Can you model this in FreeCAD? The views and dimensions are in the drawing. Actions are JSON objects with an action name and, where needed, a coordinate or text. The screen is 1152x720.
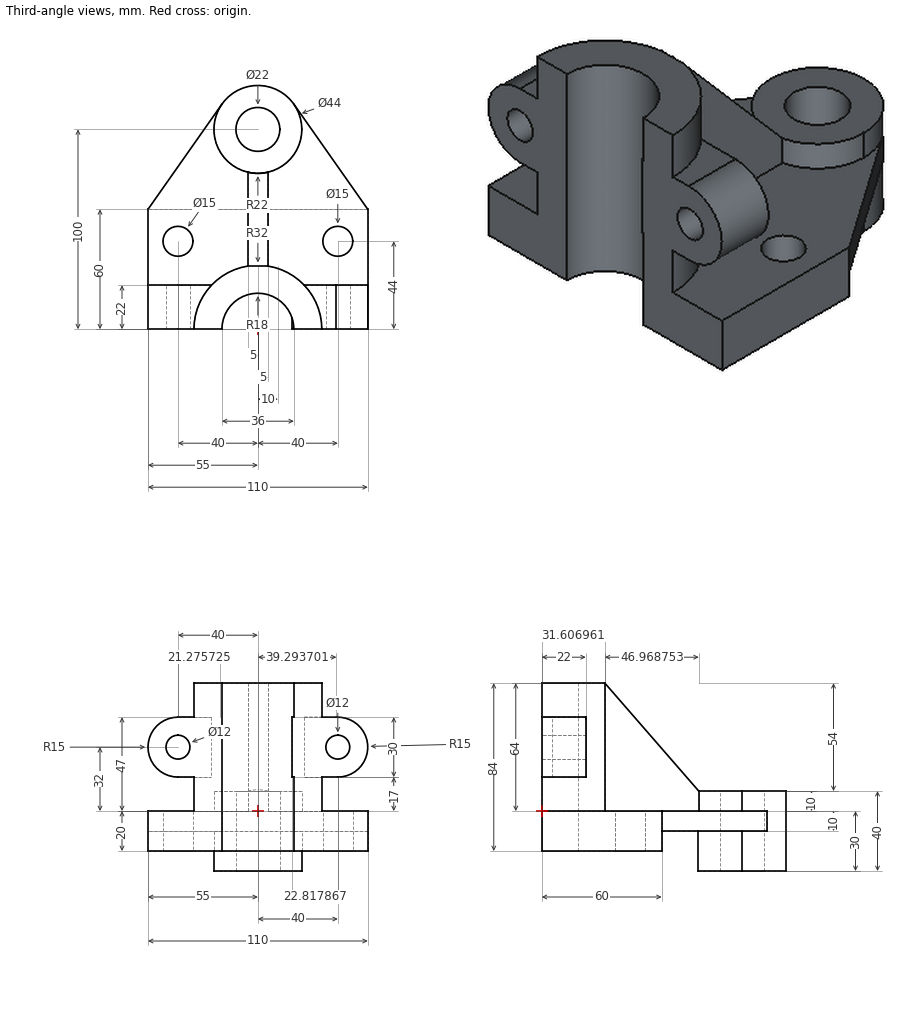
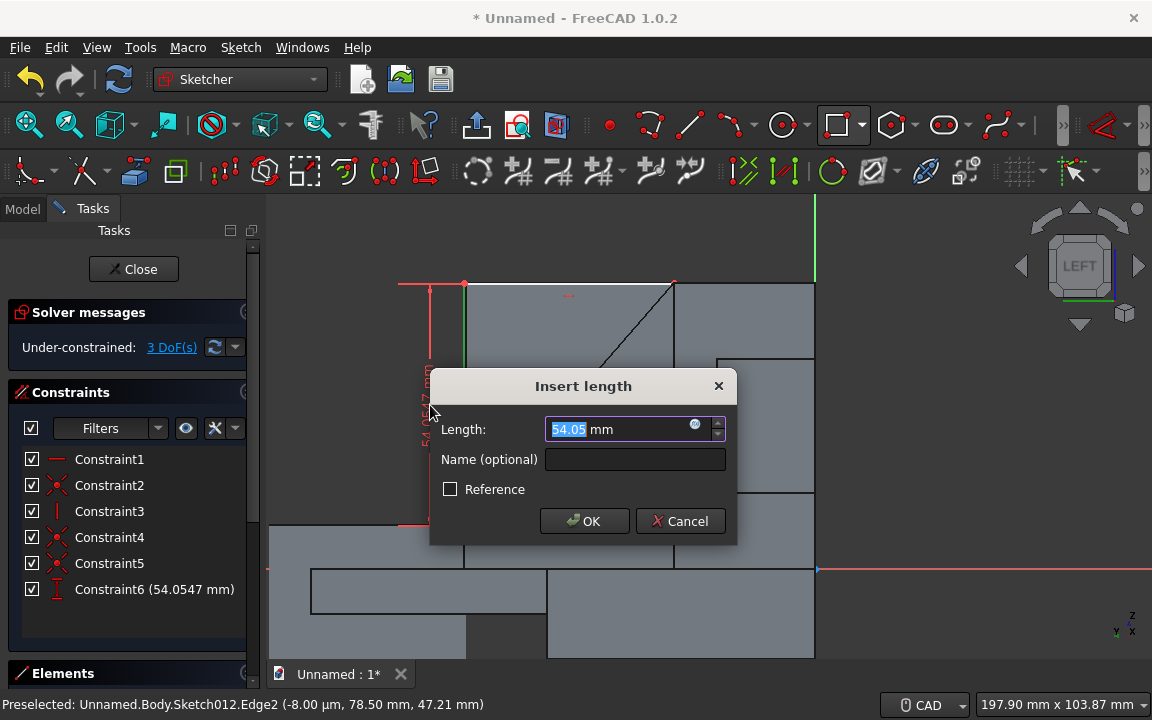
{"action": "type", "text": "54"}
{"action": "key", "text": "Return"}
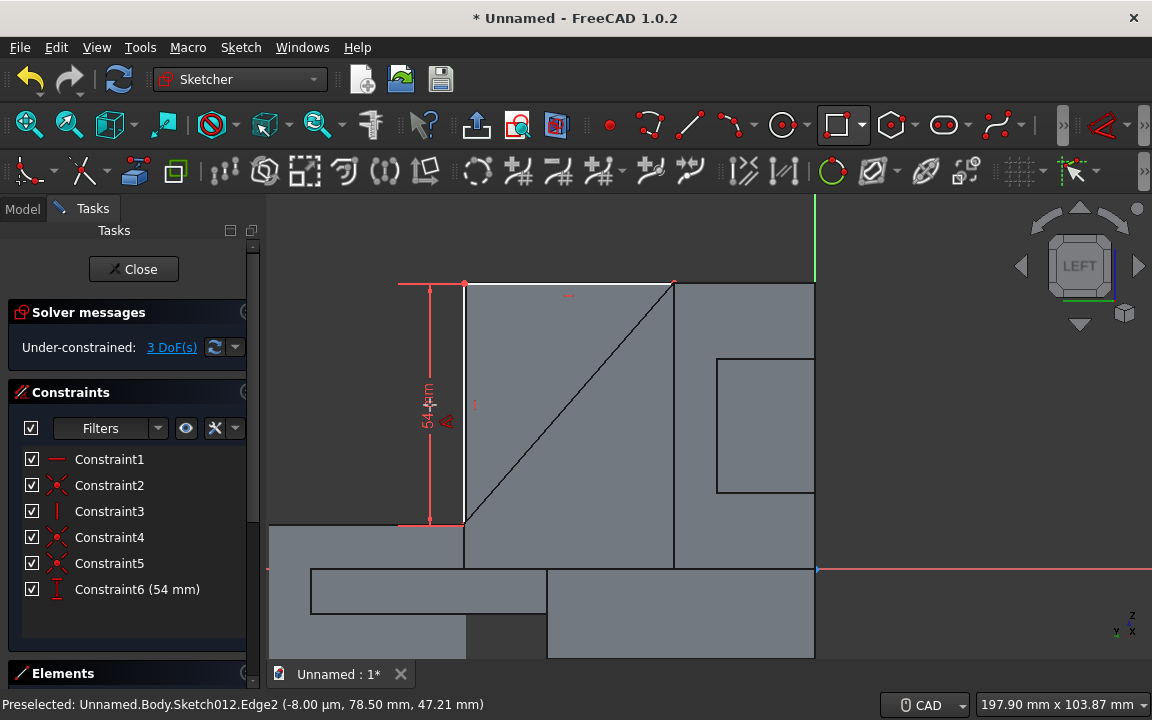
{"action": "left_click", "coordinate": [674, 284]}
{"action": "left_click", "coordinate": [849, 427]}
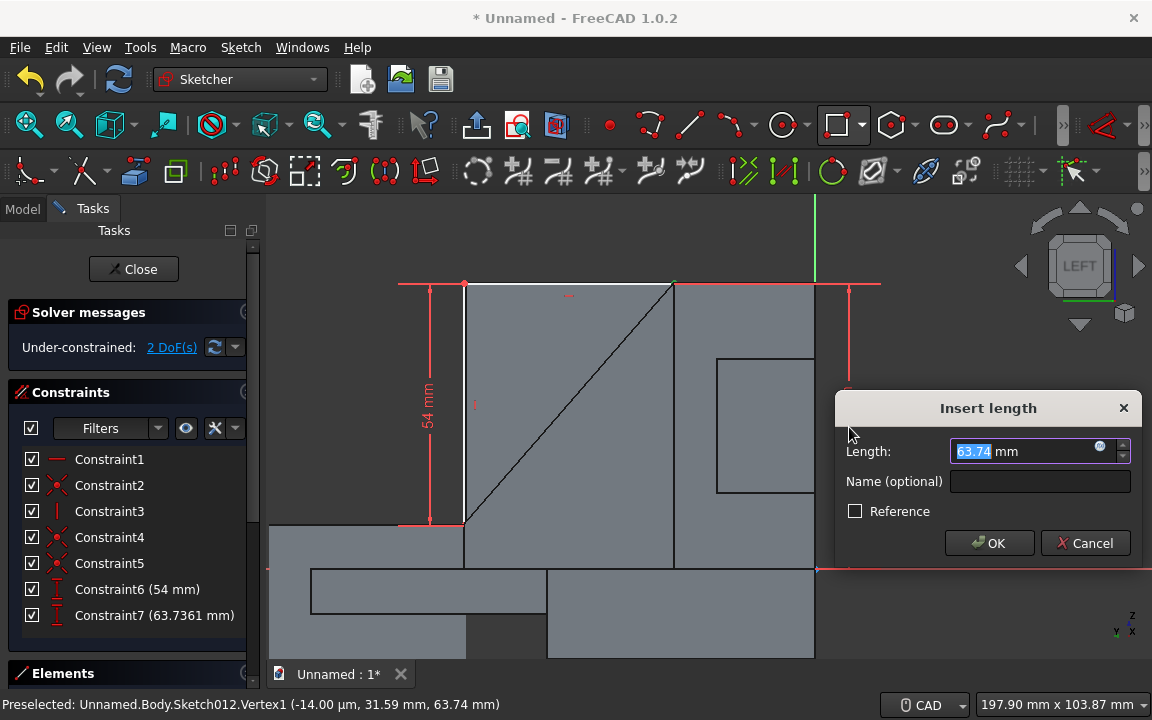
{"action": "type", "text": "64"}
{"action": "key", "text": "Return"}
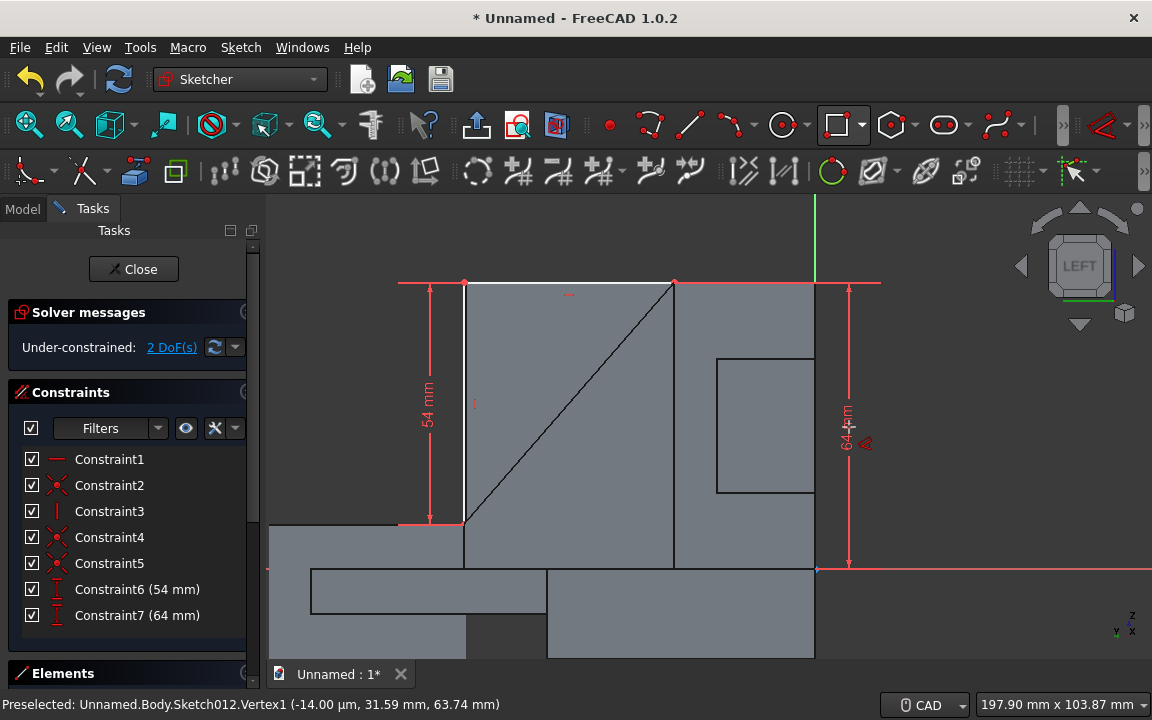
{"action": "left_click", "coordinate": [611, 283]}
{"action": "left_click", "coordinate": [569, 249]}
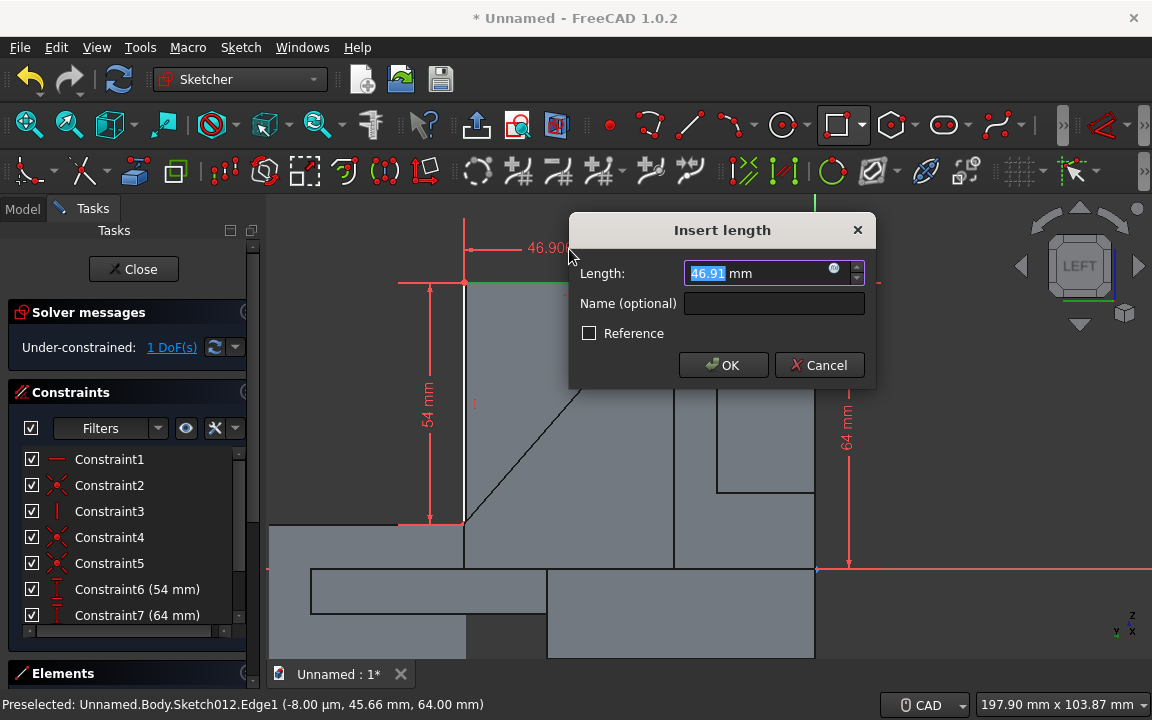
{"action": "type", "text": "46.968753"}
{"action": "key", "text": "Return"}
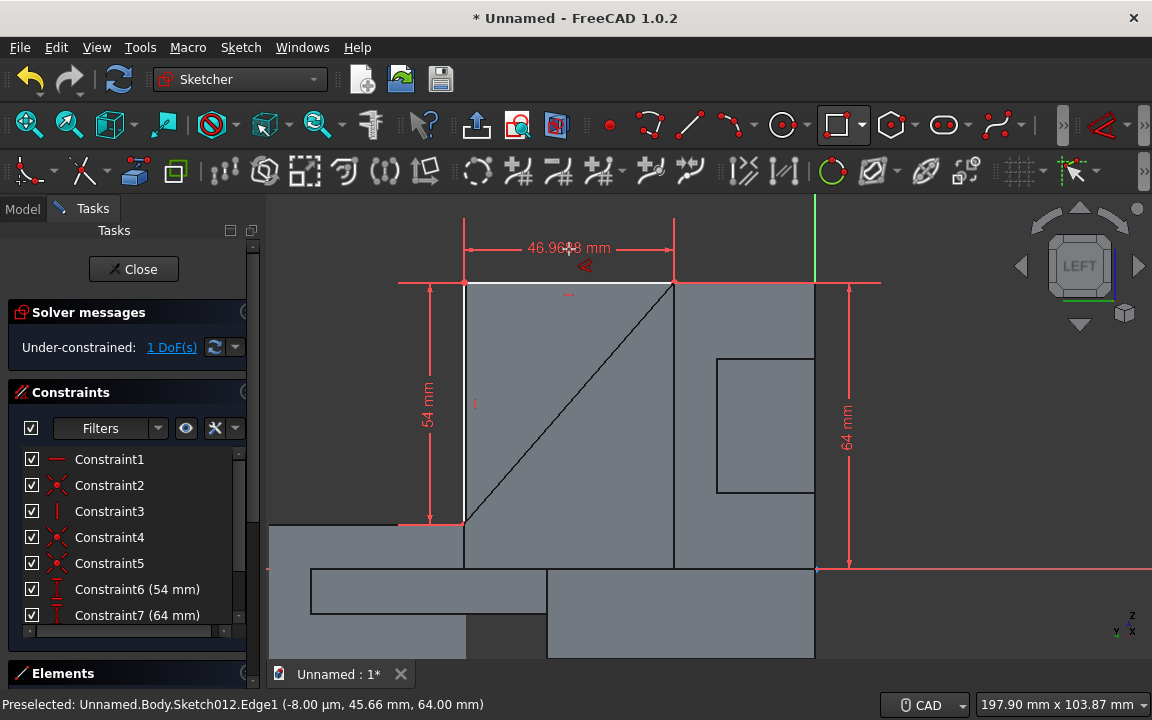
{"action": "left_click", "coordinate": [674, 283]}
{"action": "left_click", "coordinate": [745, 603]}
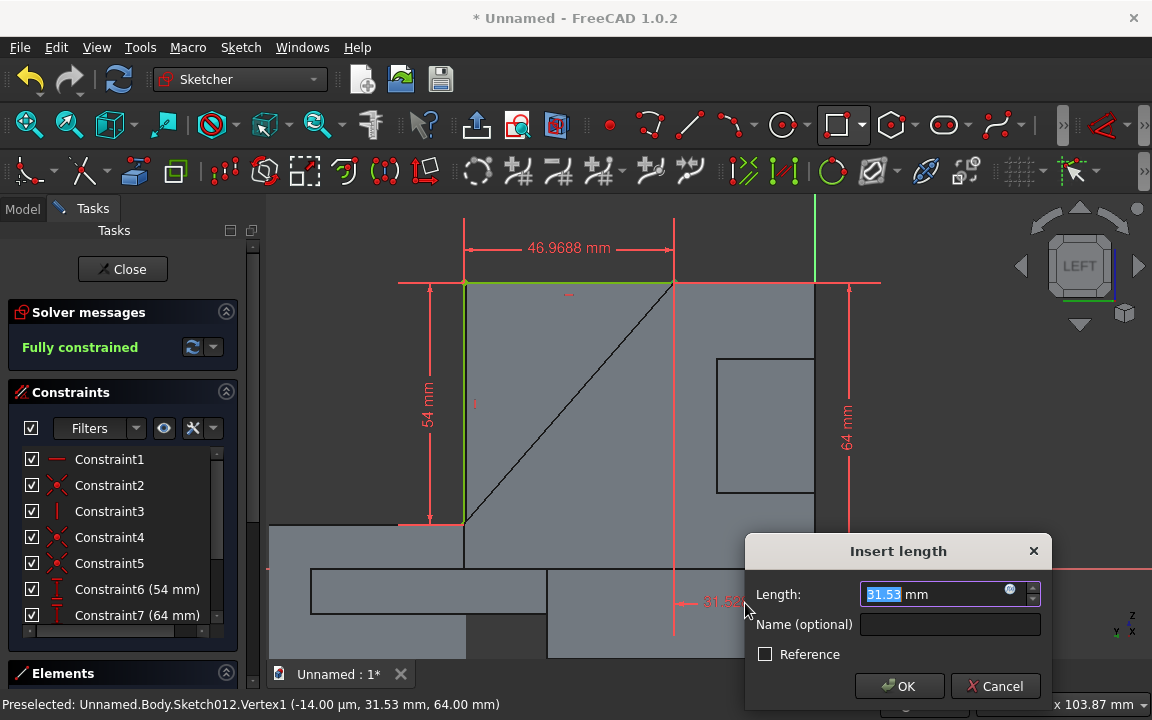
{"action": "type", "text": "31.606961"}
{"action": "key", "text": "Return"}
{"action": "key", "text": "Escape"}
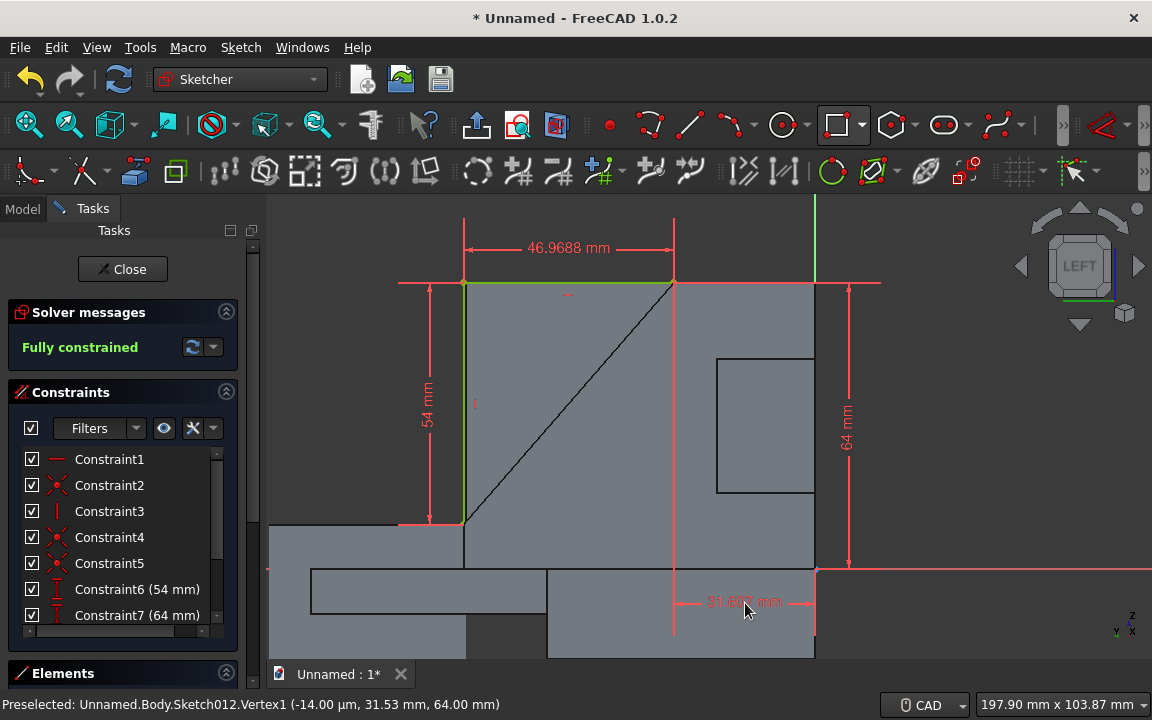
{"action": "left_click", "coordinate": [123, 269]}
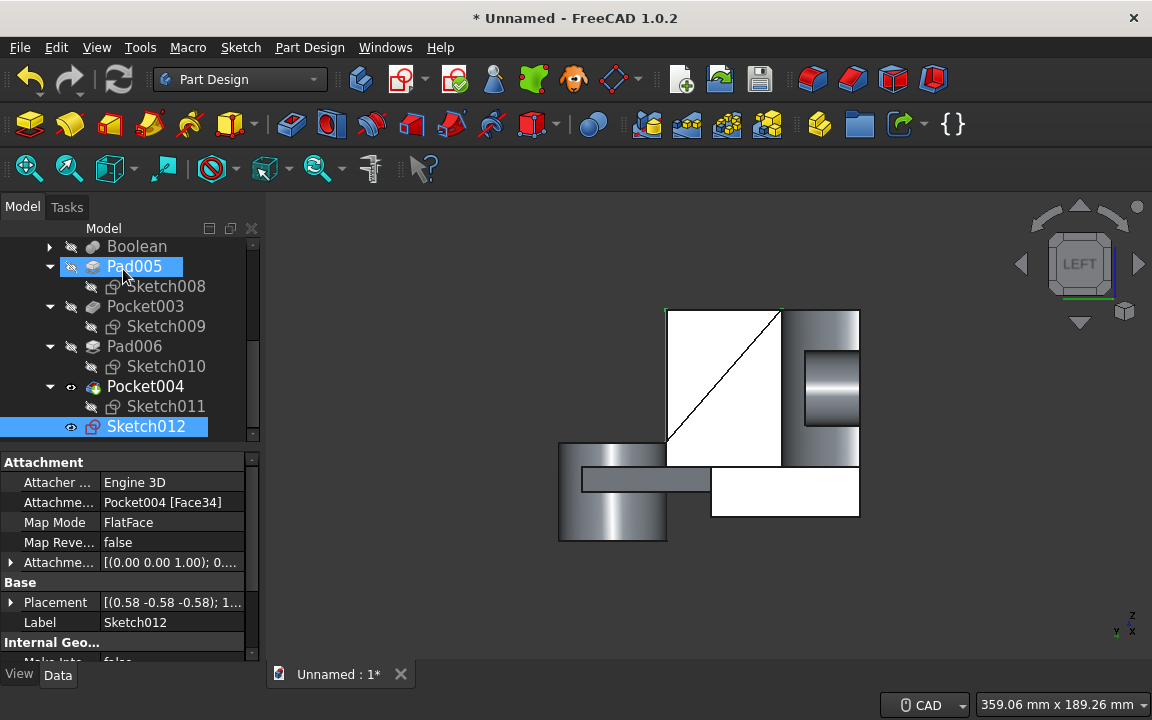
{"action": "left_click", "coordinate": [292, 124]}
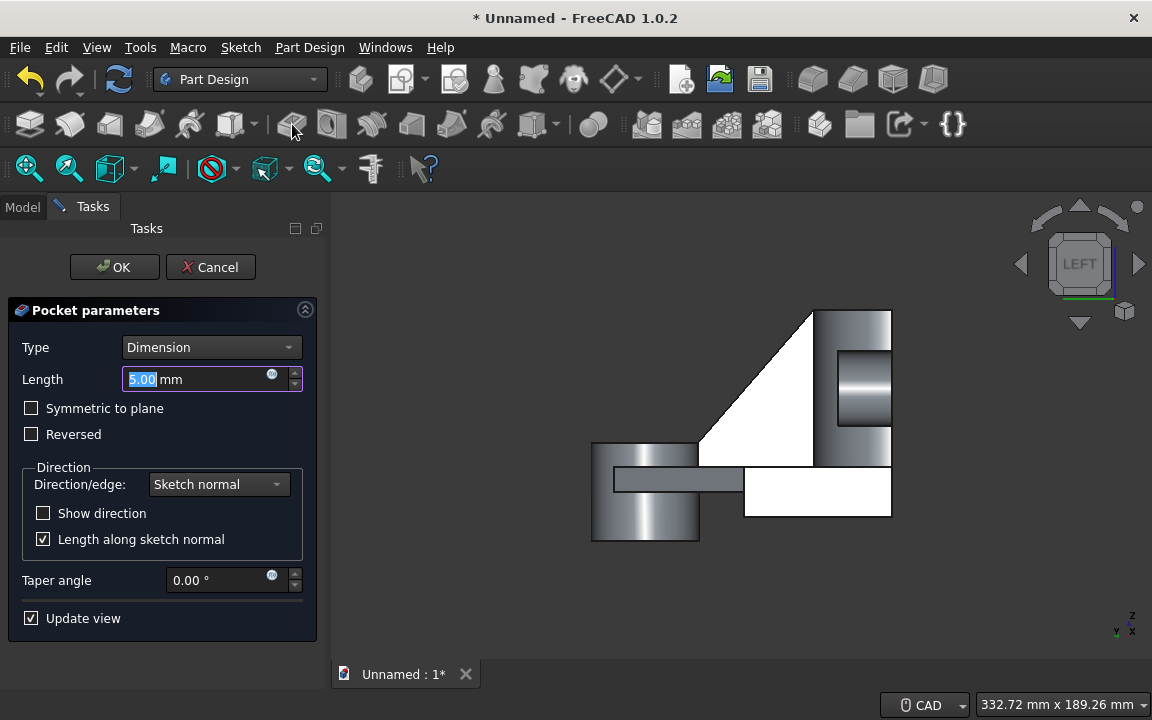
{"action": "type", "text": "10"}
{"action": "key", "text": "Tab"}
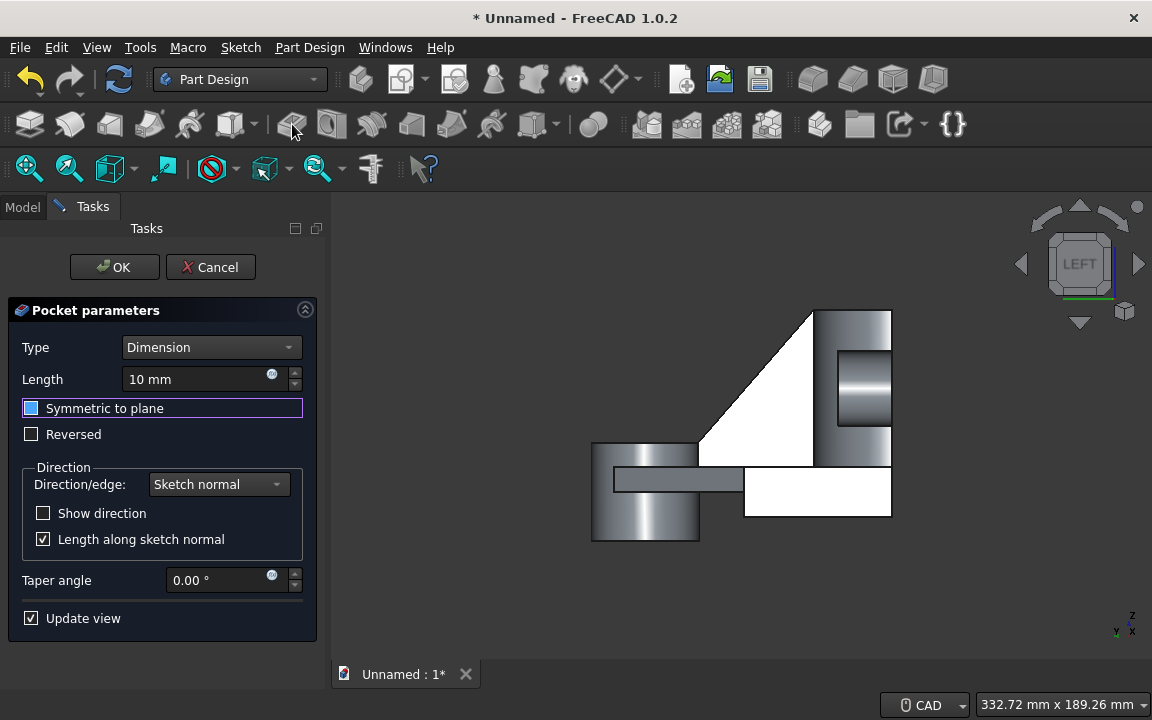
{"action": "left_click", "coordinate": [115, 267]}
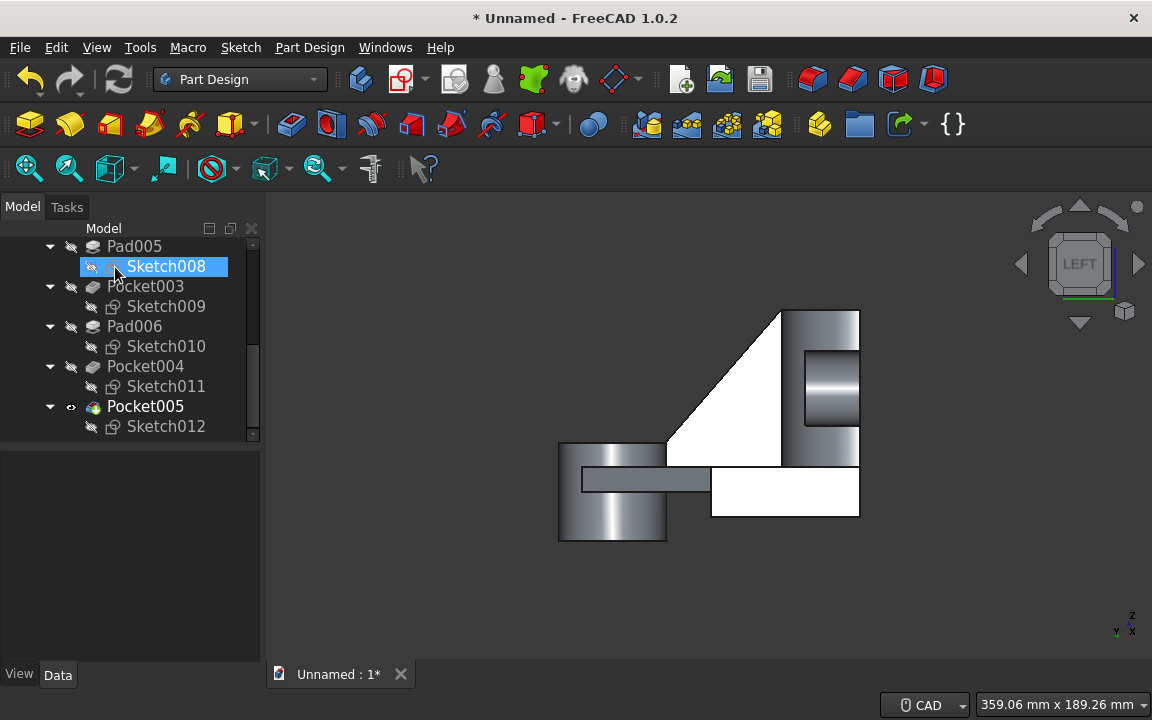
{"action": "left_click", "coordinate": [402, 80]}